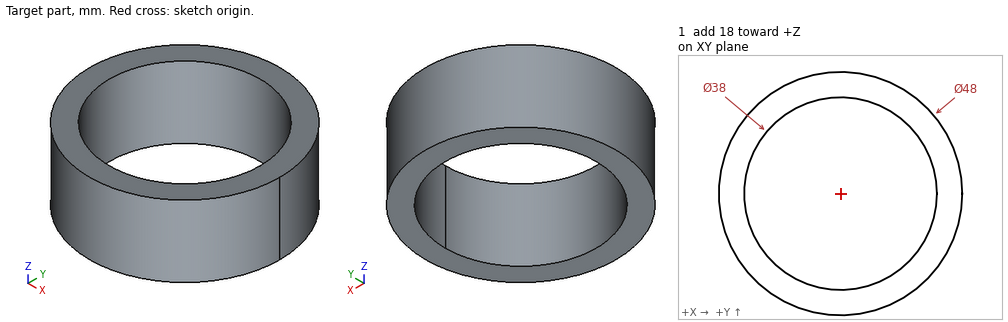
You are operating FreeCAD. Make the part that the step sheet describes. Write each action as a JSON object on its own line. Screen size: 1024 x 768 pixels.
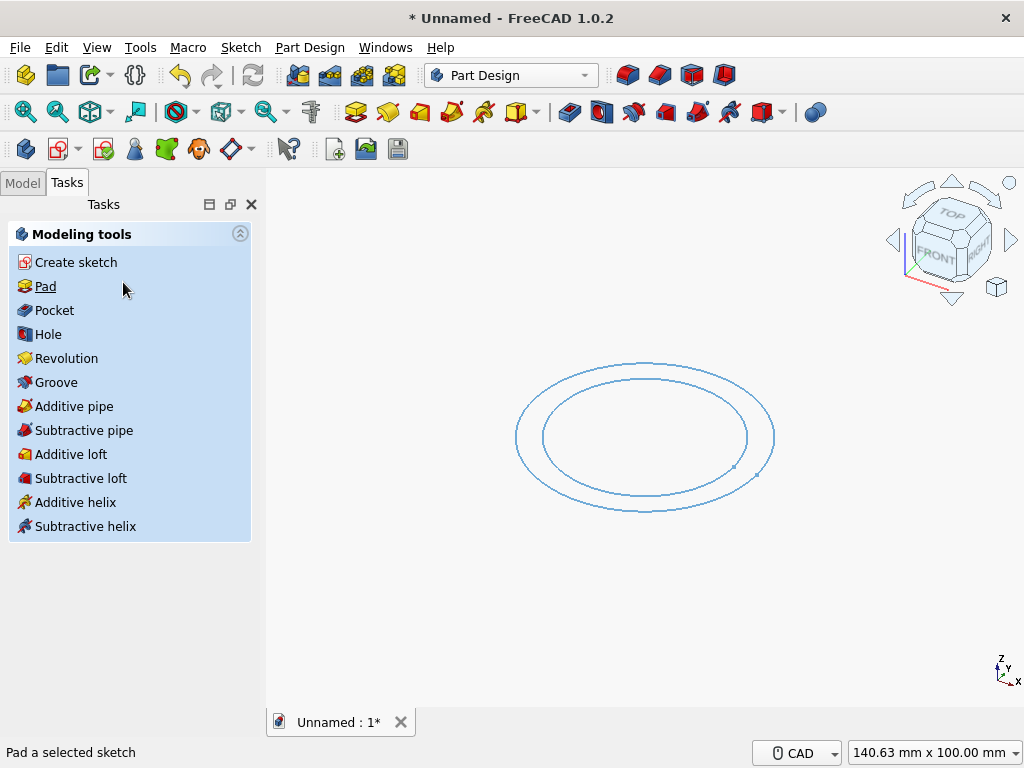
{"action": "left_click", "coordinate": [356, 112]}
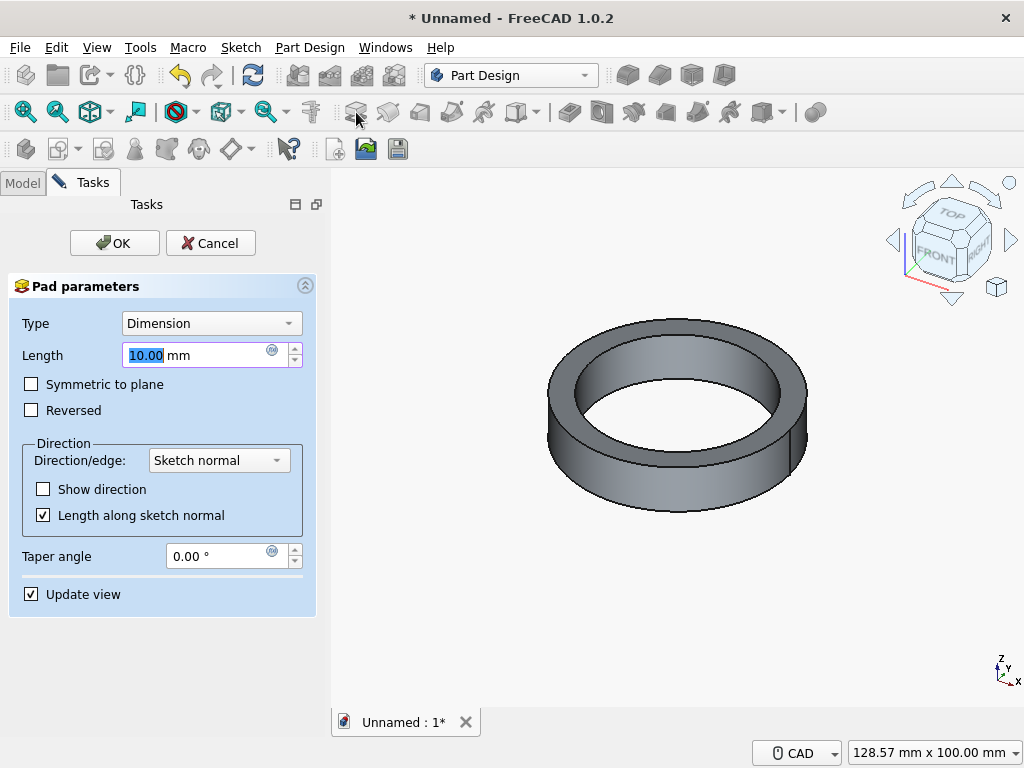
{"action": "type", "text": "18"}
{"action": "key", "text": "Tab"}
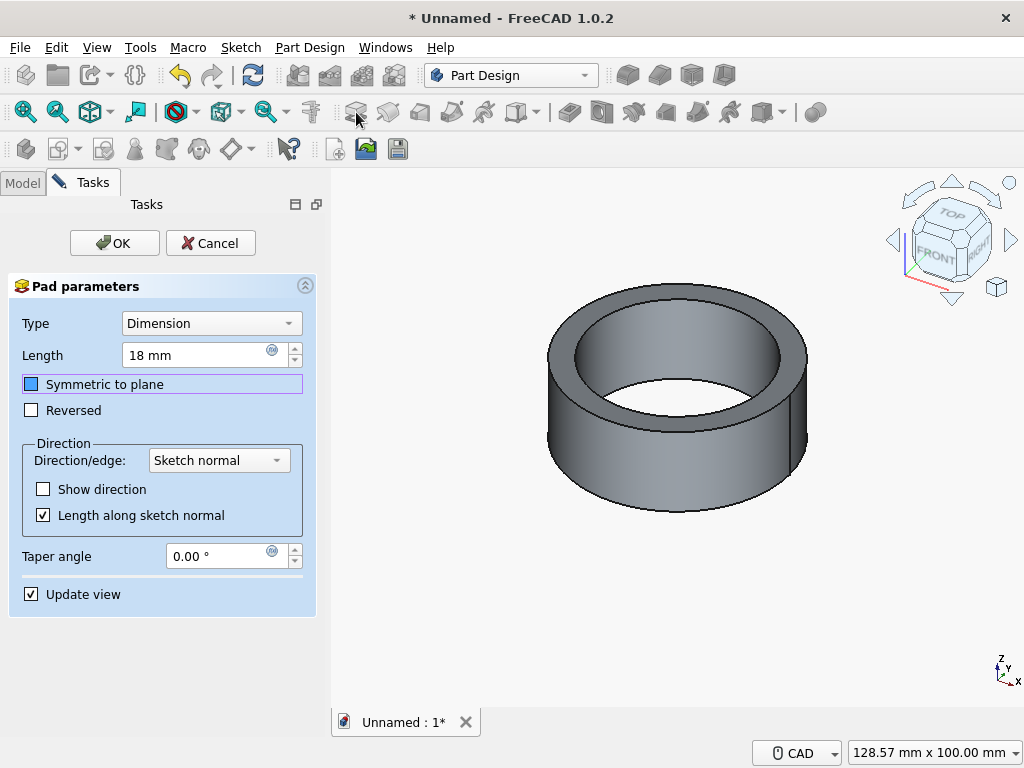
{"action": "left_click", "coordinate": [115, 243]}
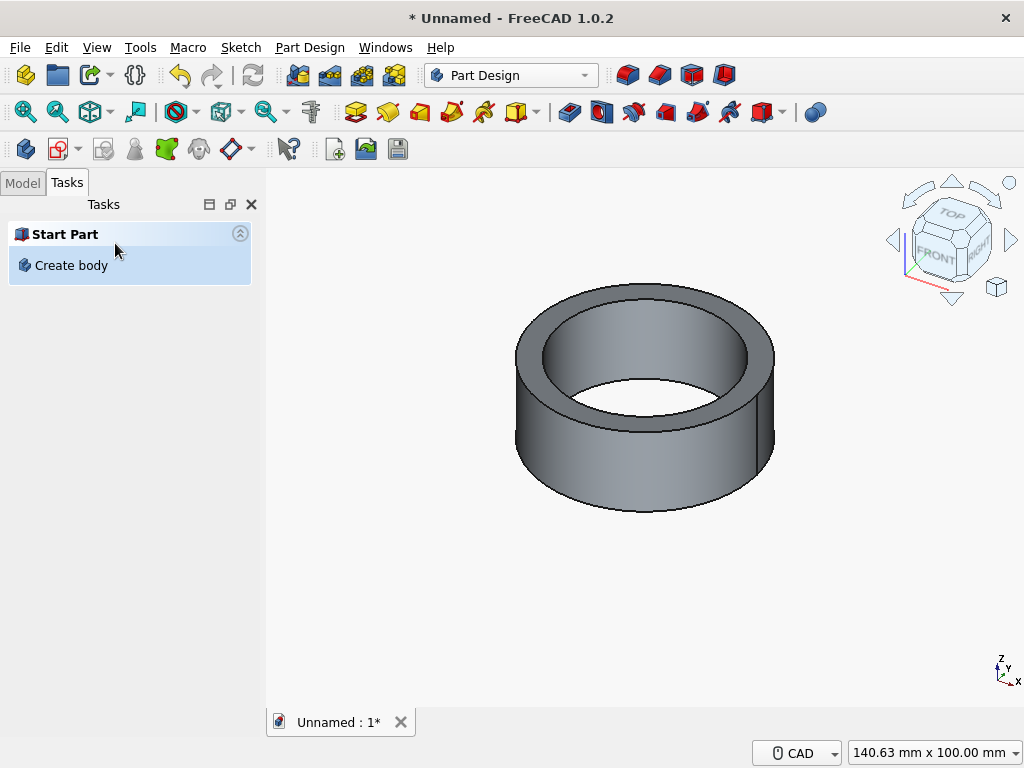
{"action": "key", "text": "0"}